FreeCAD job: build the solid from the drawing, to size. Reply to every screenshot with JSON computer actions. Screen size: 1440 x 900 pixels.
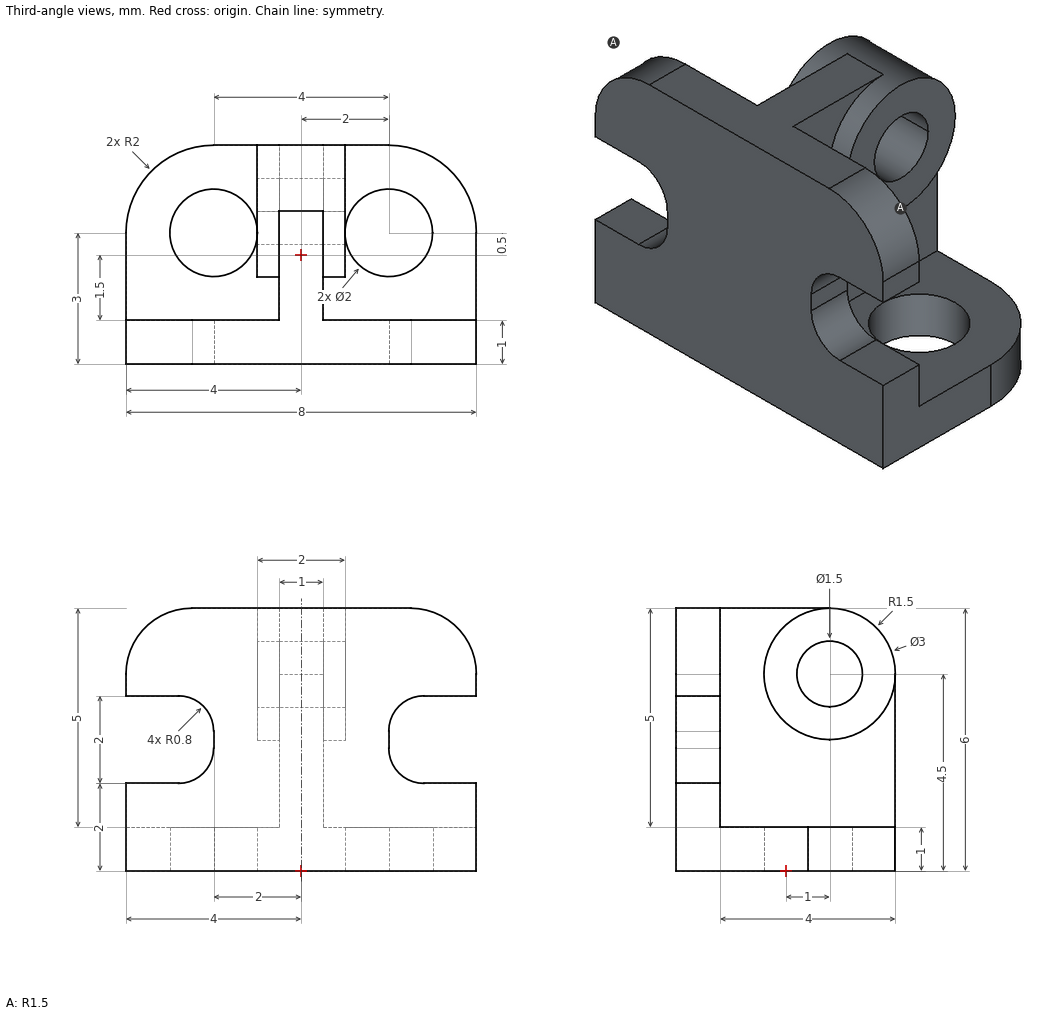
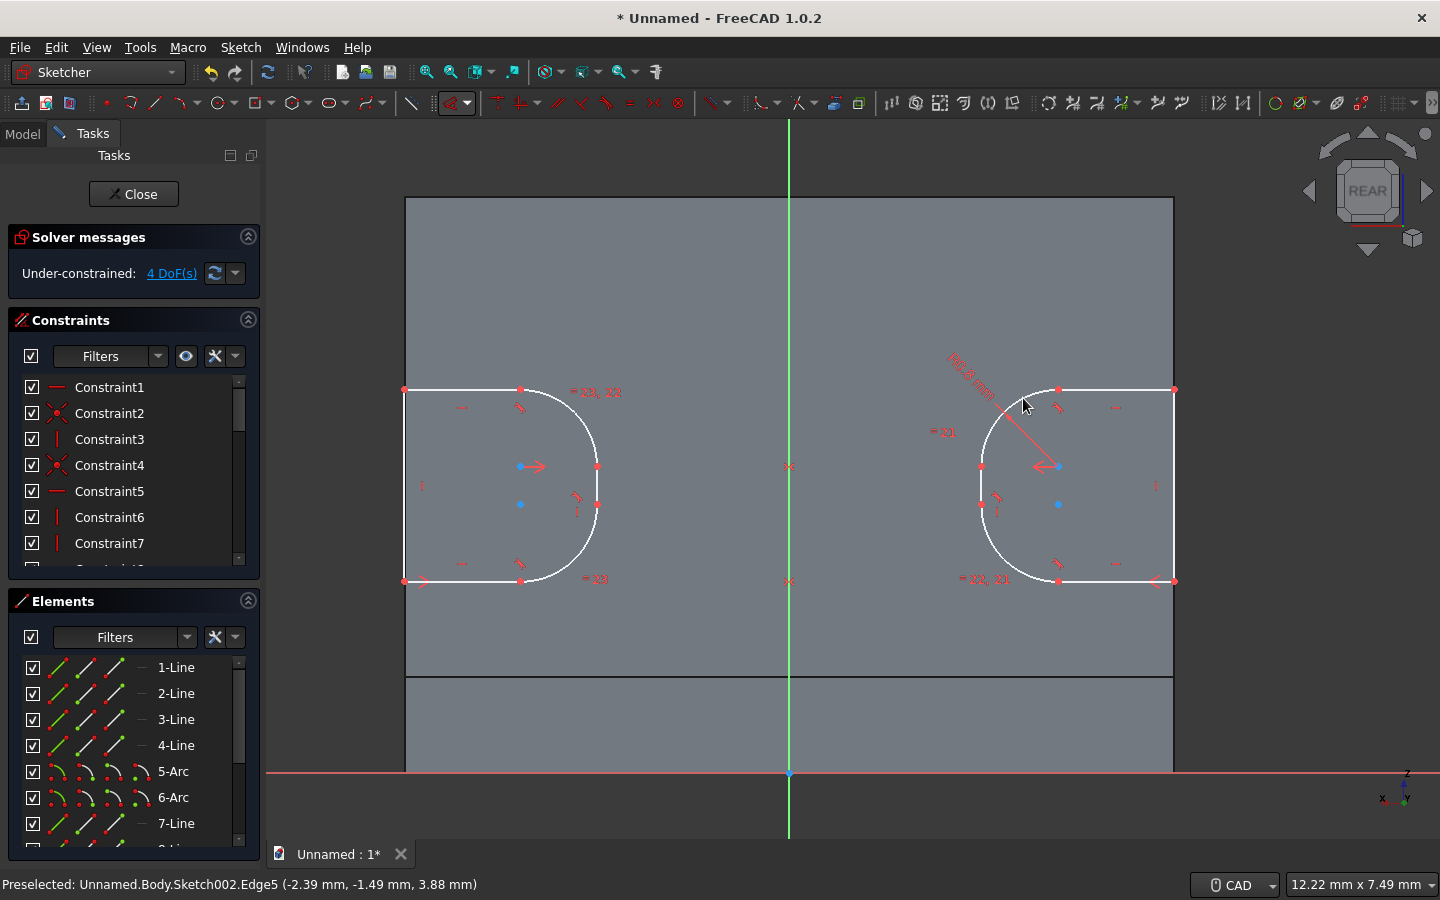
{"action": "left_click", "coordinate": [1174, 524]}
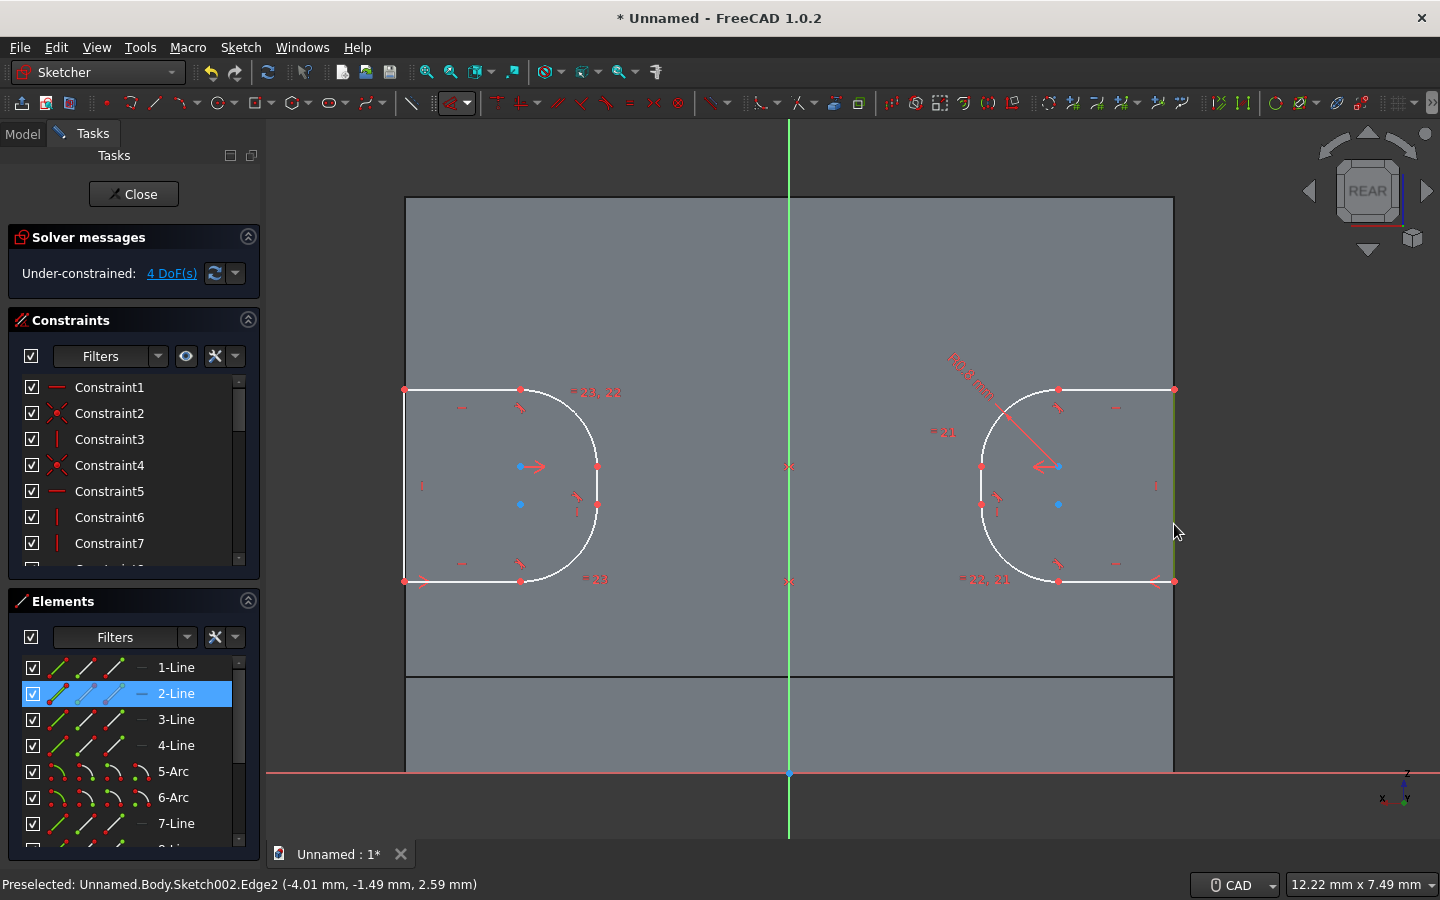
{"action": "key", "text": "i"}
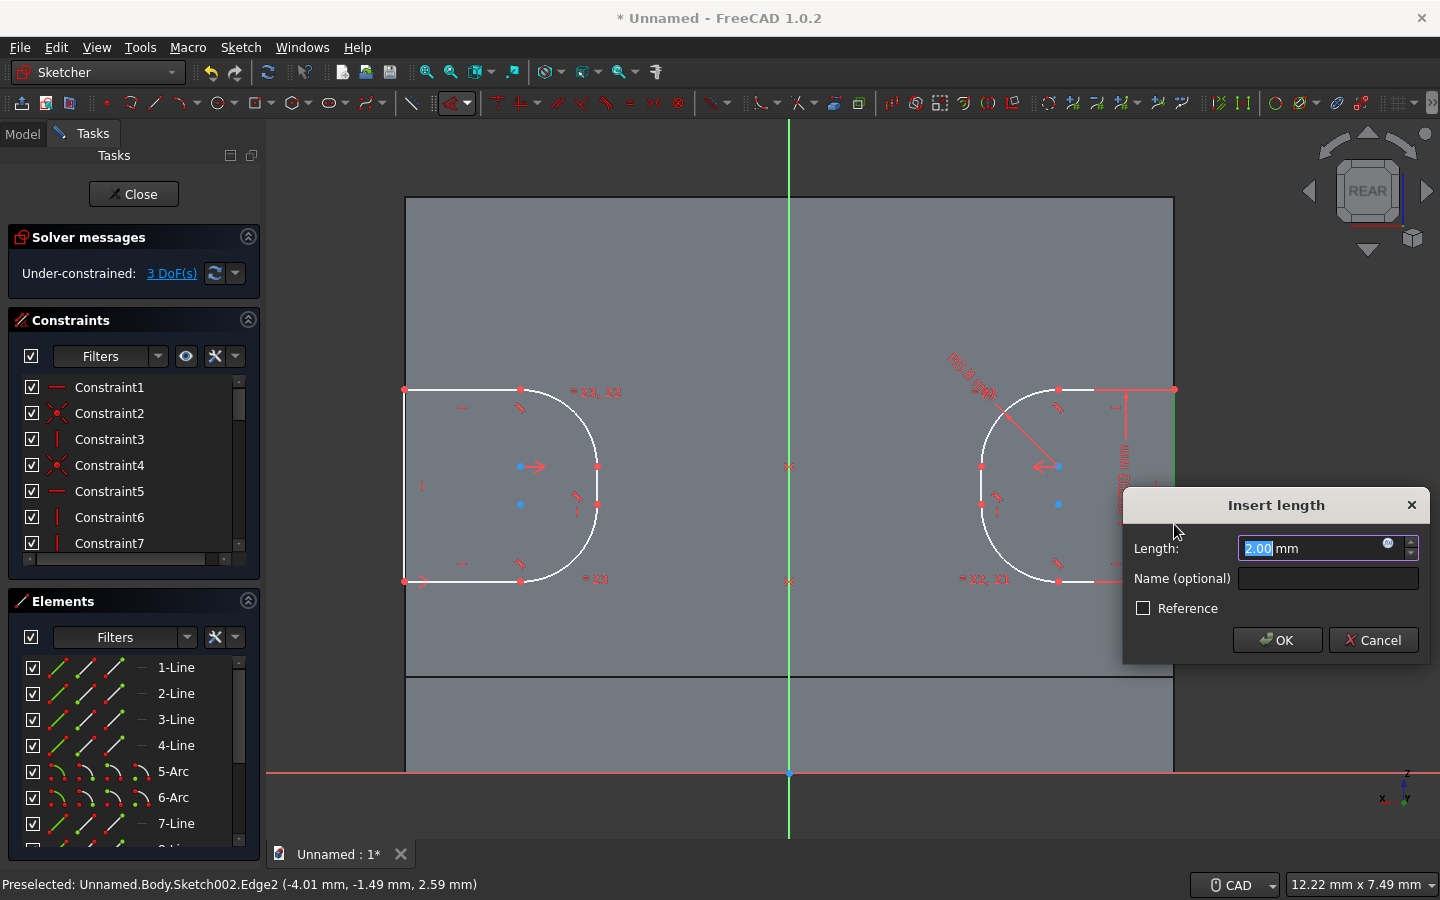
{"action": "type", "text": "2"}
{"action": "key", "text": "Return"}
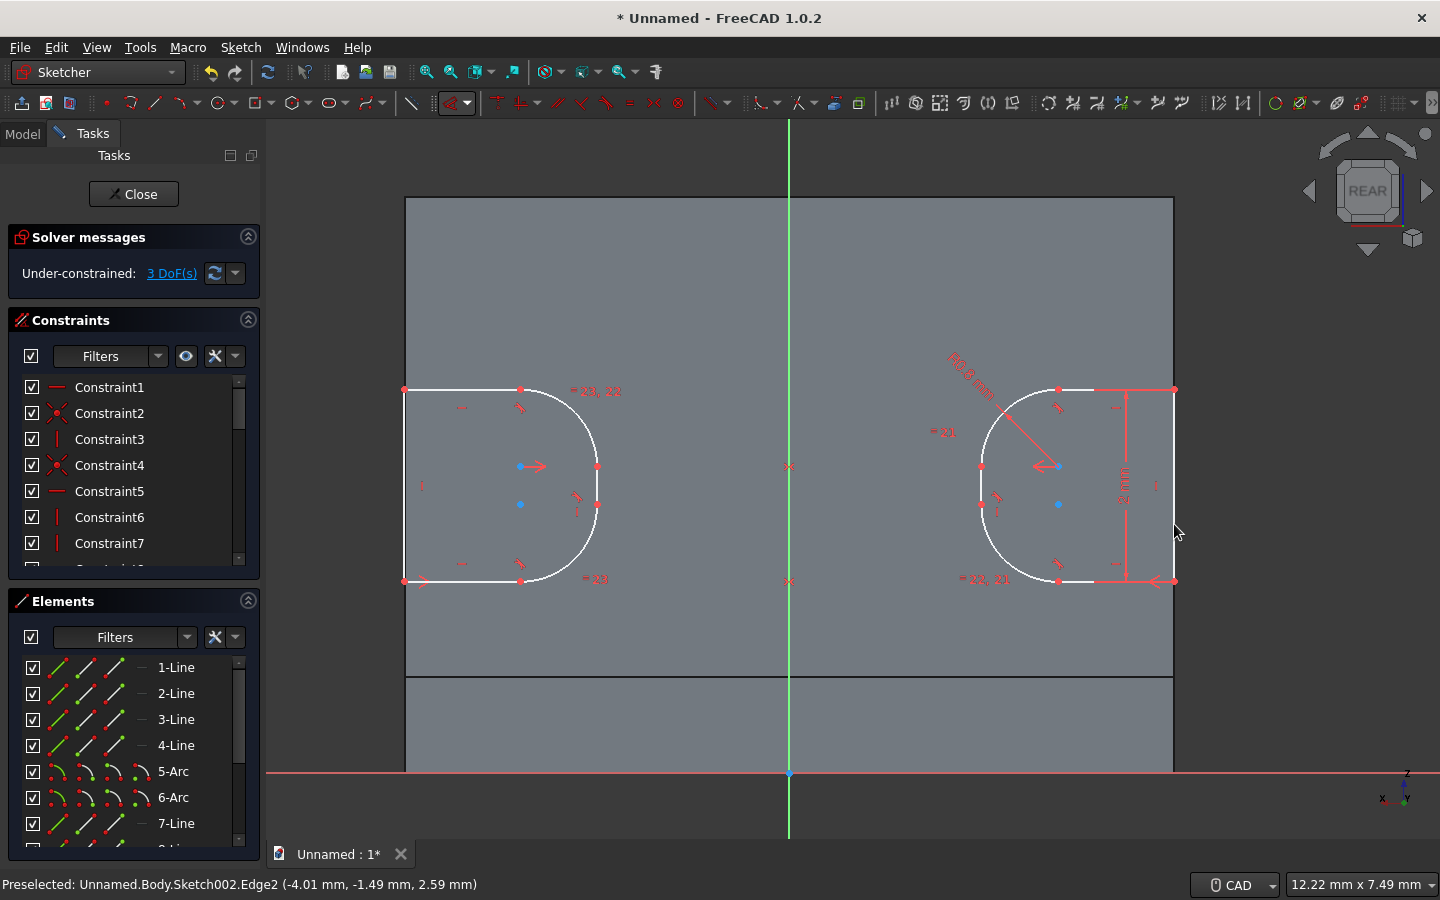
{"action": "left_click", "coordinate": [1058, 582]}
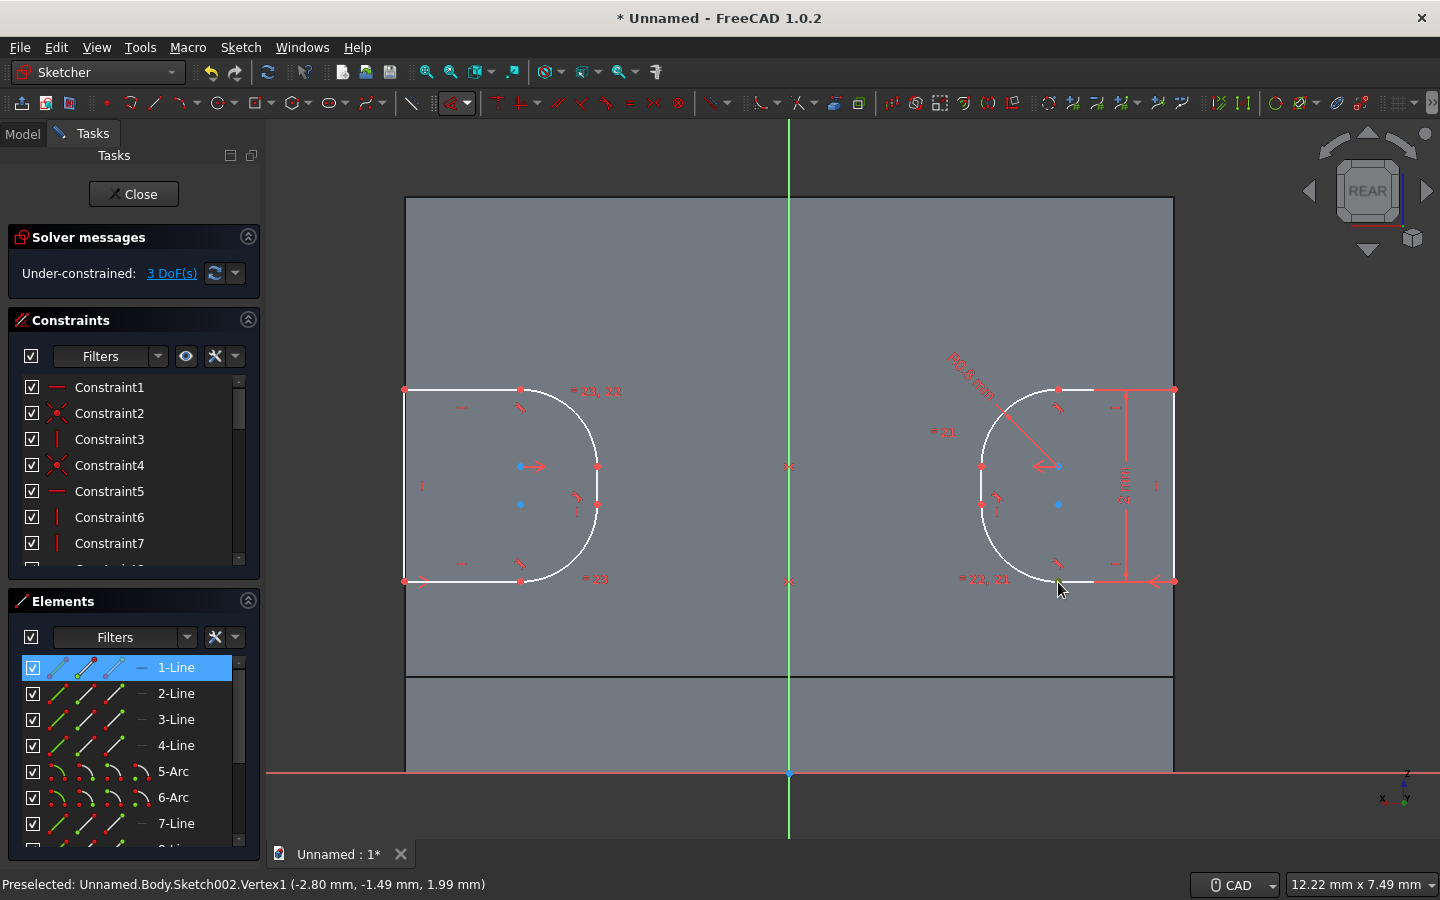
{"action": "key", "text": "i"}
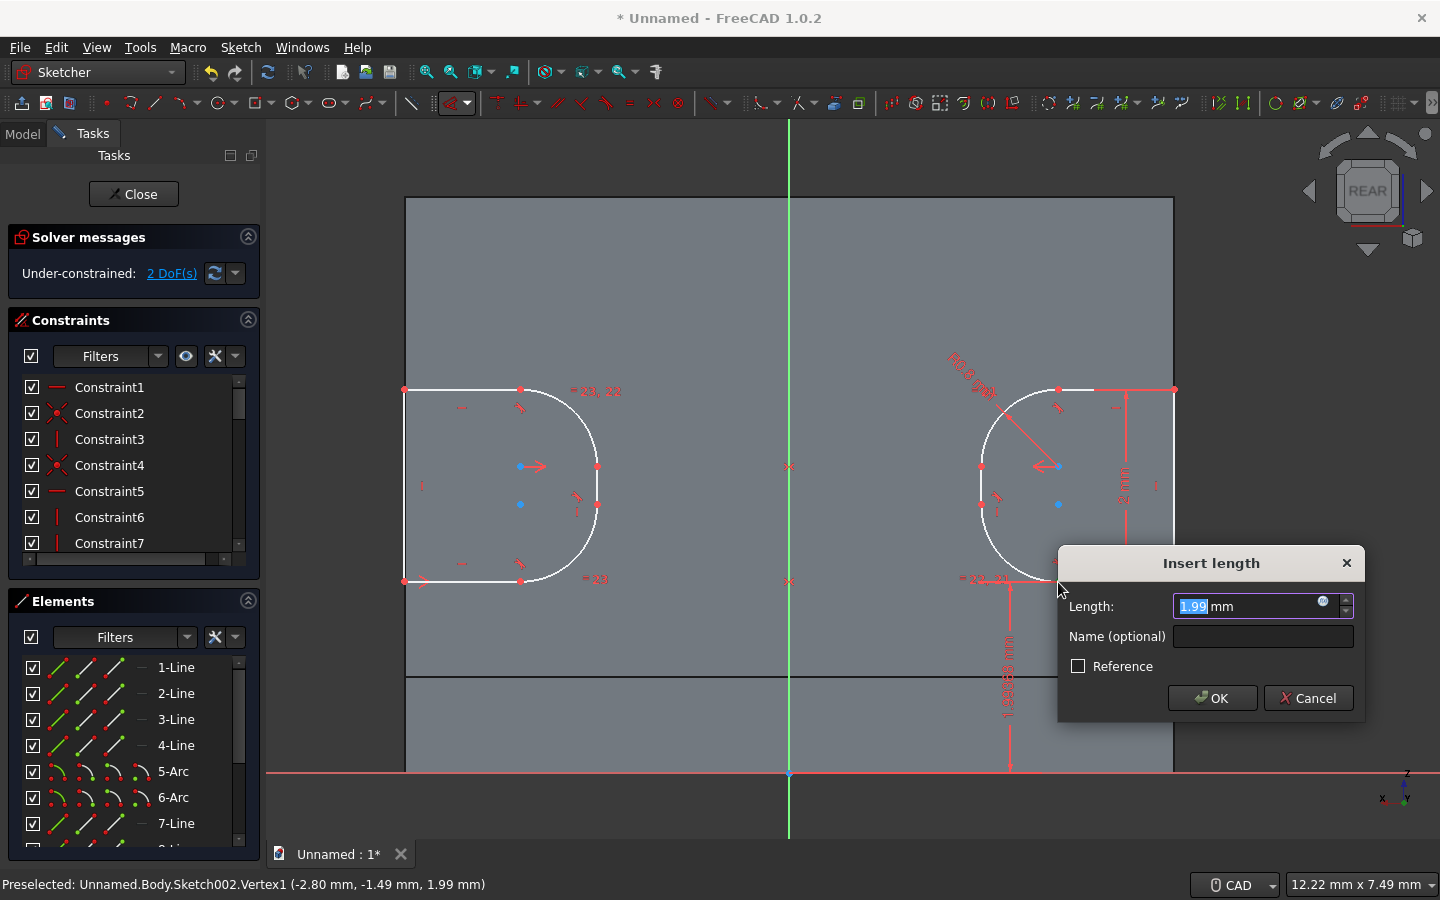
{"action": "type", "text": "2"}
{"action": "key", "text": "Return"}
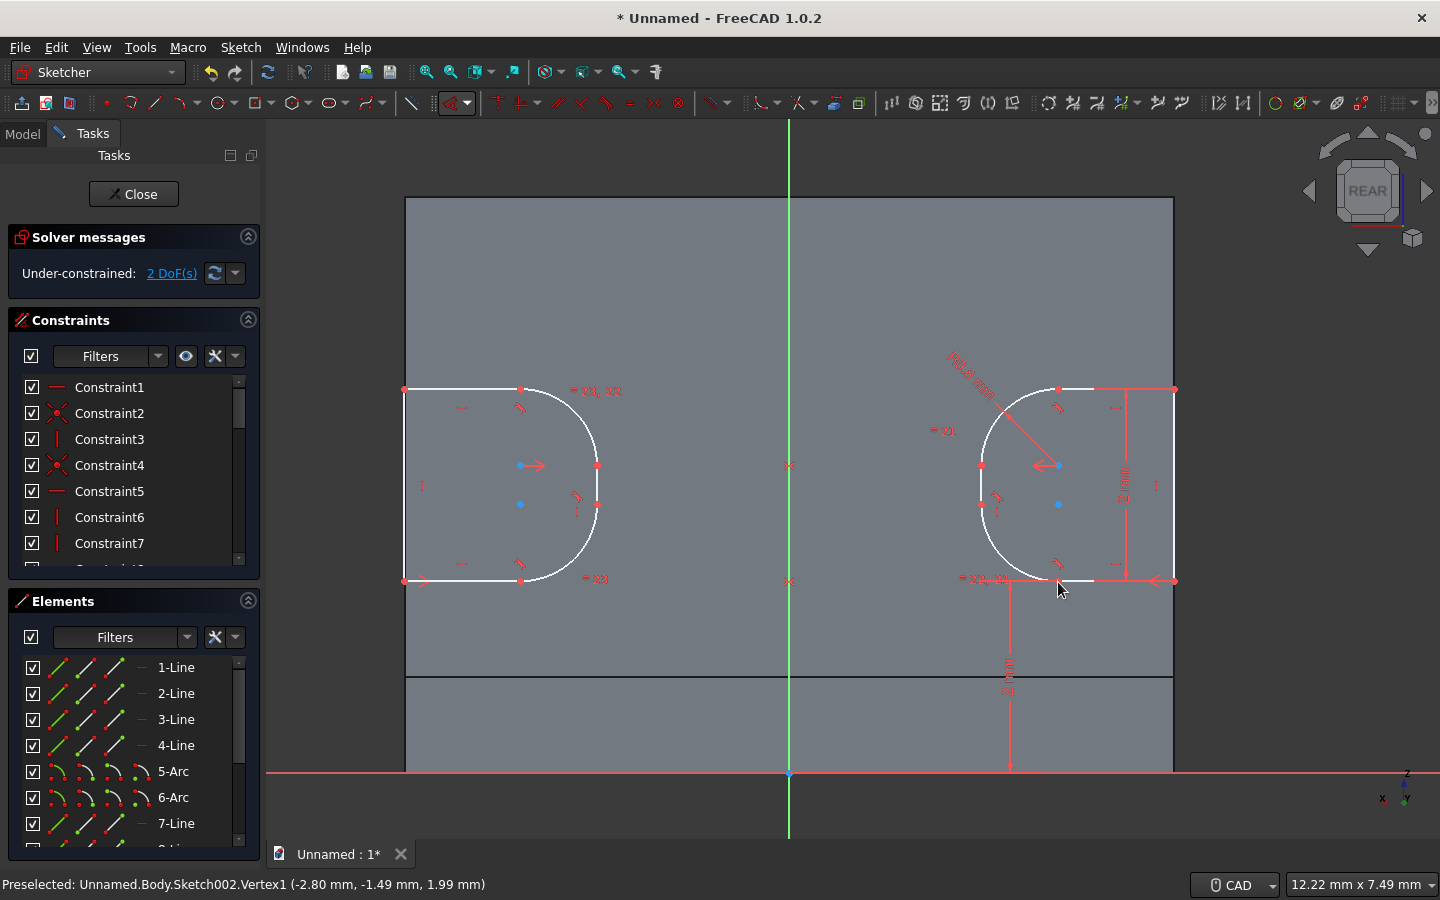
{"action": "left_click", "coordinate": [1174, 581]}